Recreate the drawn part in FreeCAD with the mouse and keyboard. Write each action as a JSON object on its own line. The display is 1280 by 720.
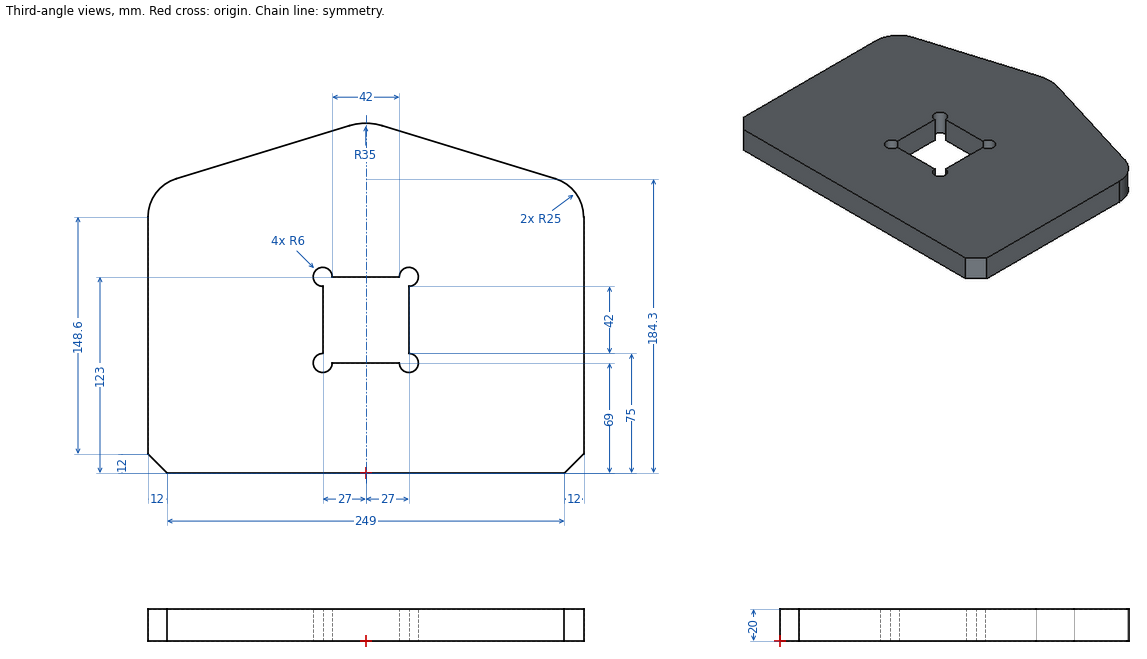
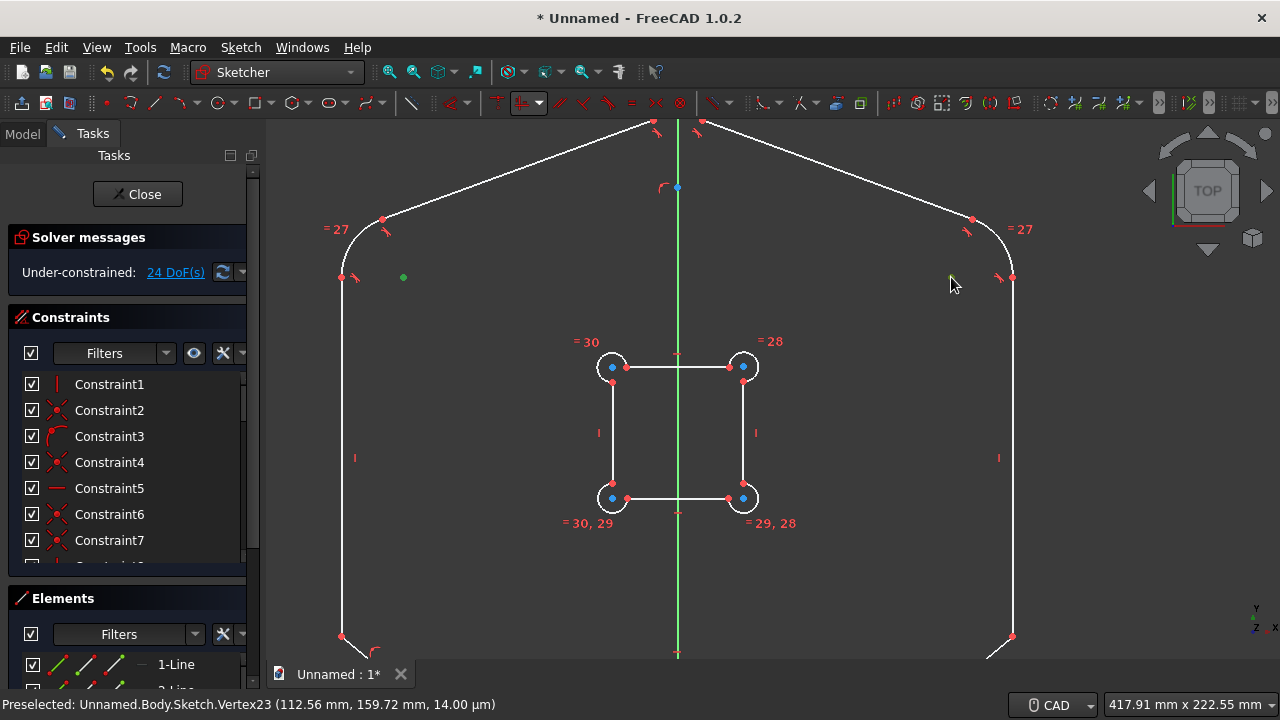
{"action": "left_click", "coordinate": [678, 596]}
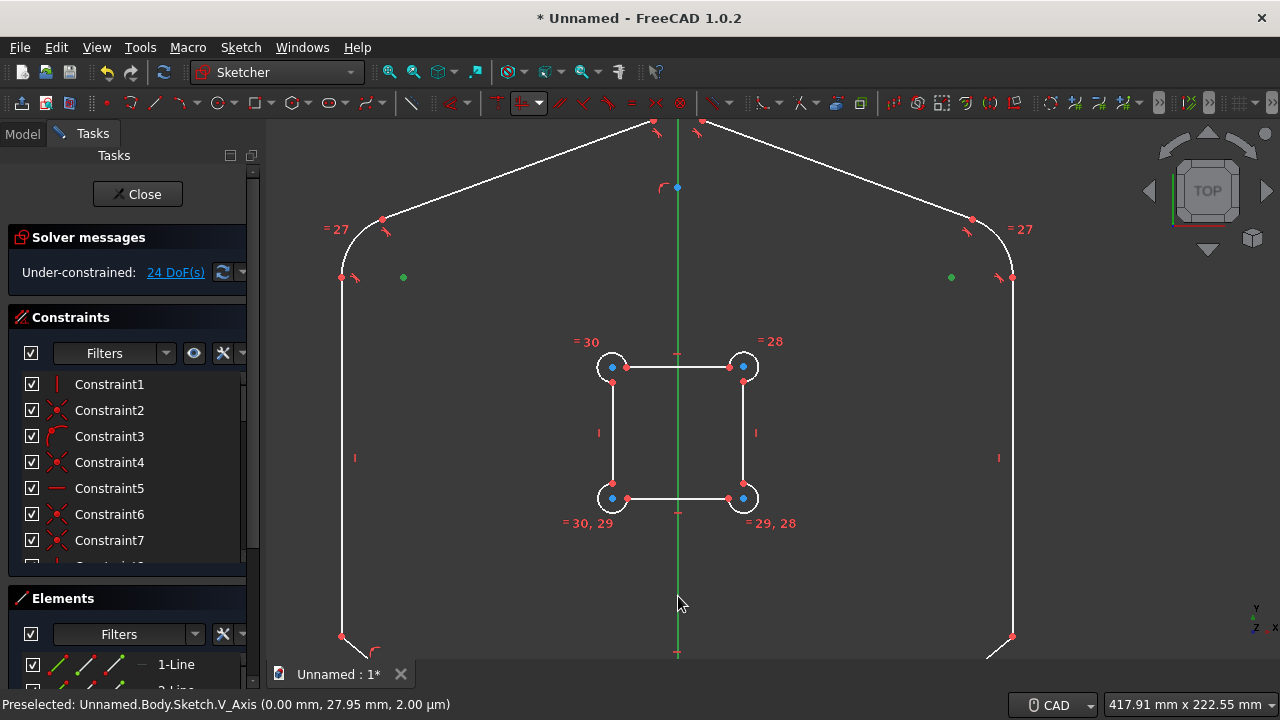
{"action": "left_click", "coordinate": [656, 104]}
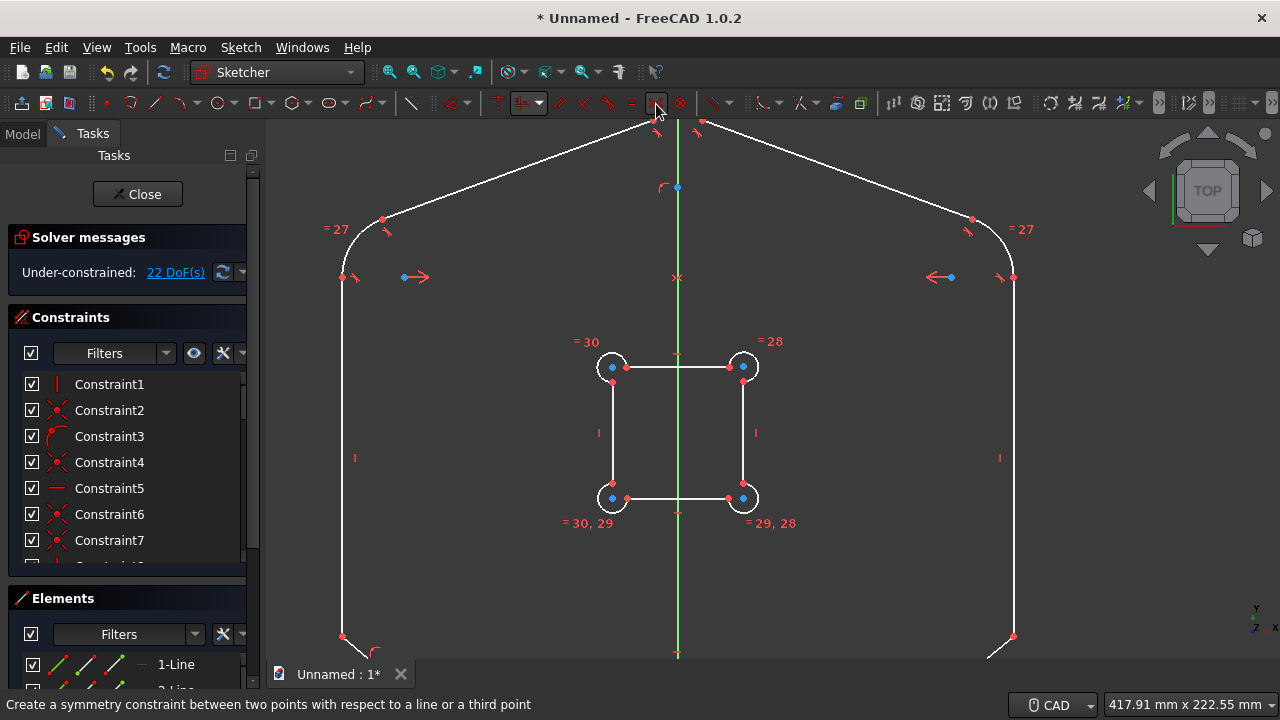
{"action": "left_click", "coordinate": [744, 498]}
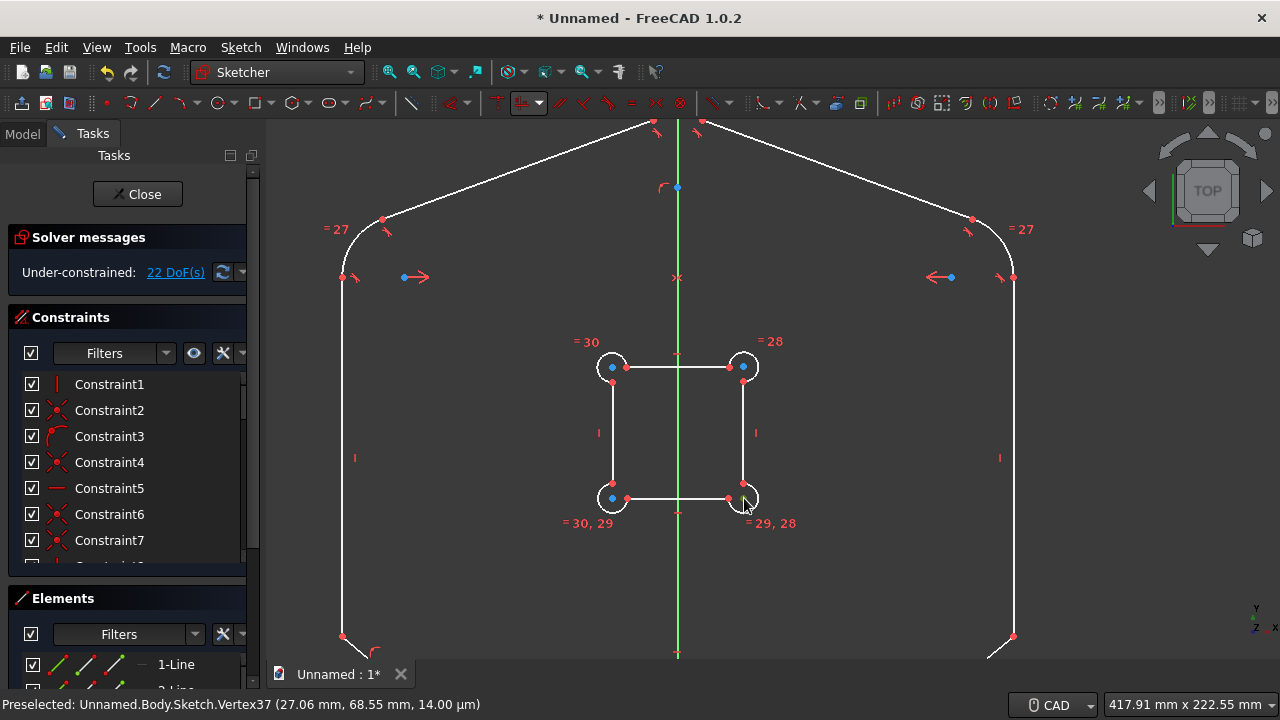
{"action": "left_click", "coordinate": [613, 498]}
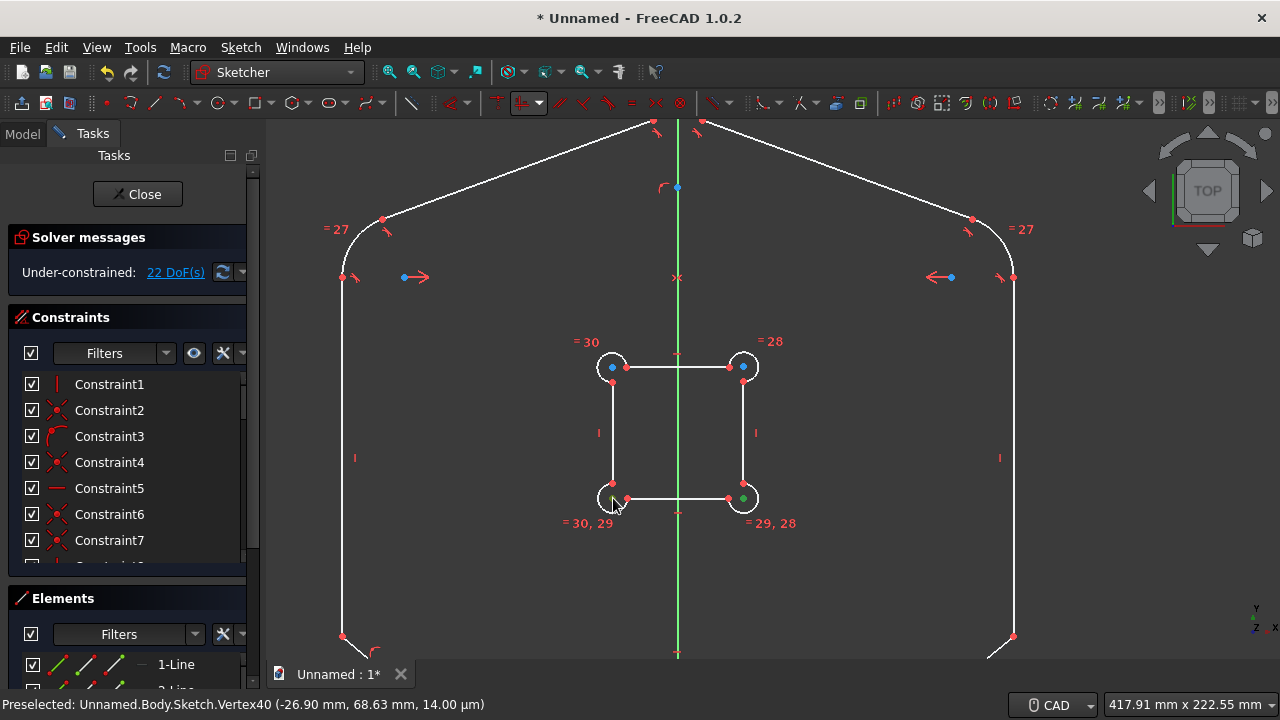
{"action": "left_click", "coordinate": [678, 596]}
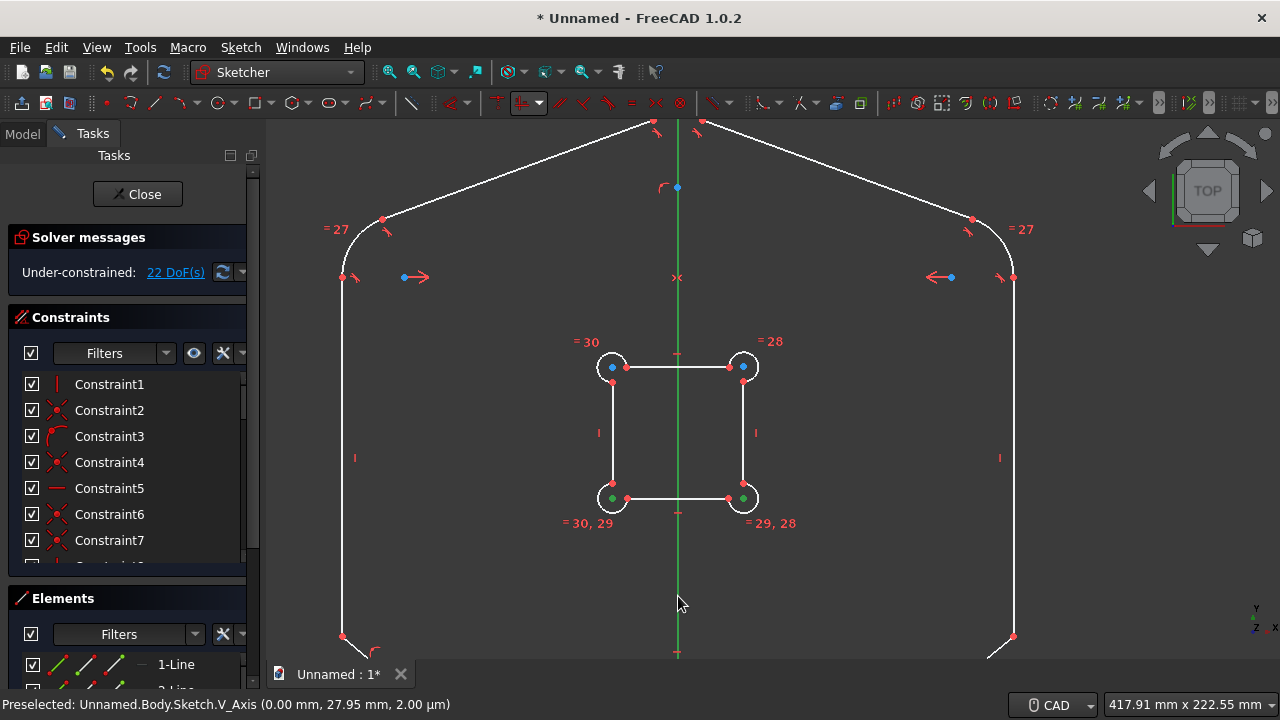
{"action": "left_click", "coordinate": [656, 104]}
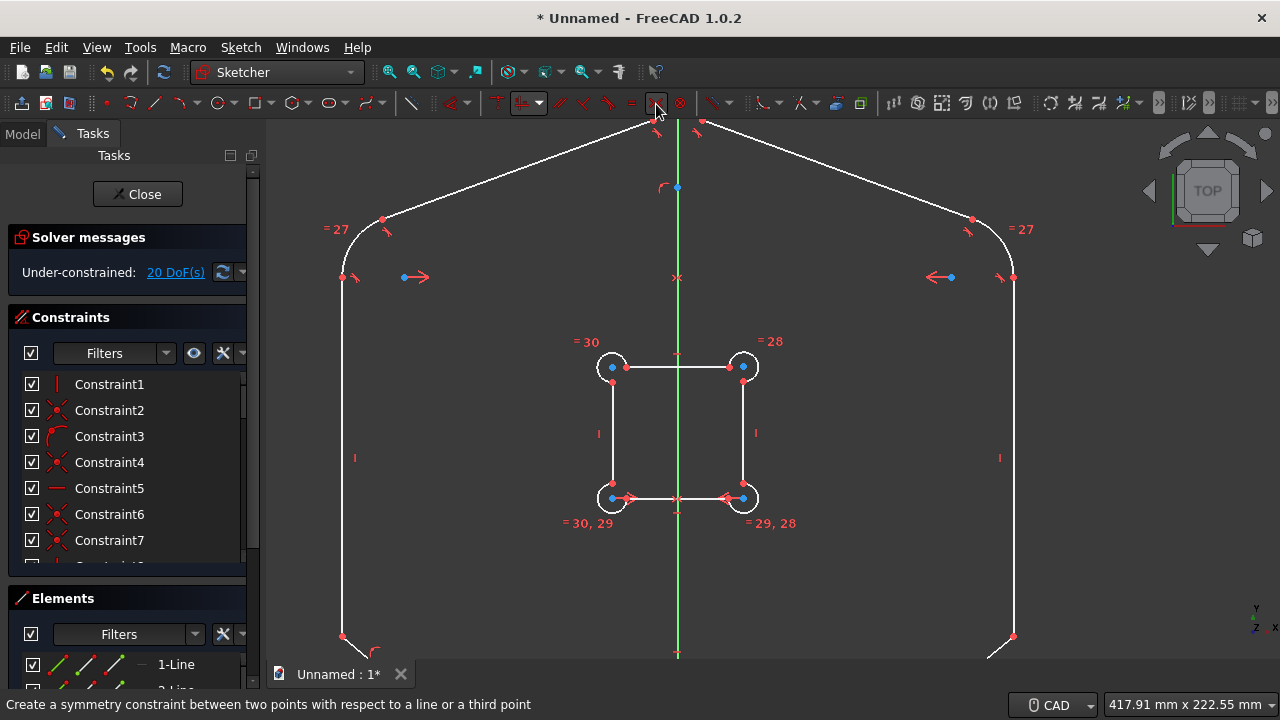
{"action": "left_click", "coordinate": [744, 367]}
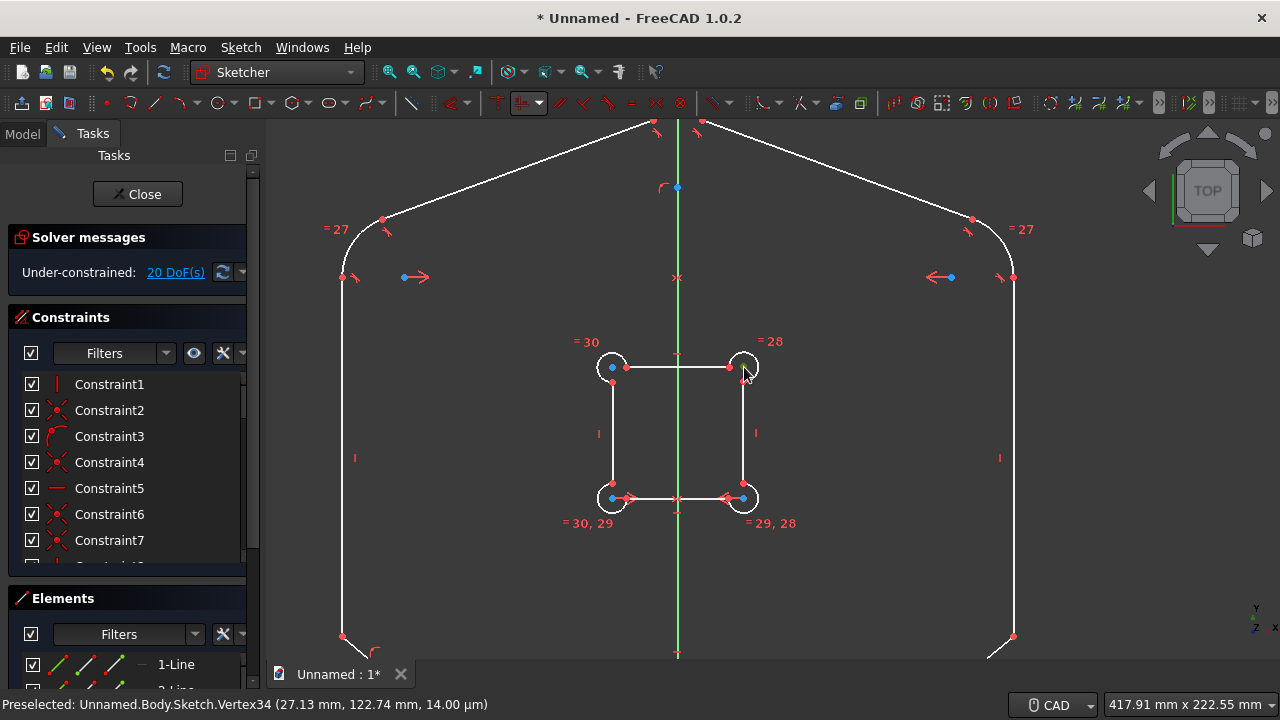
{"action": "left_click", "coordinate": [612, 368]}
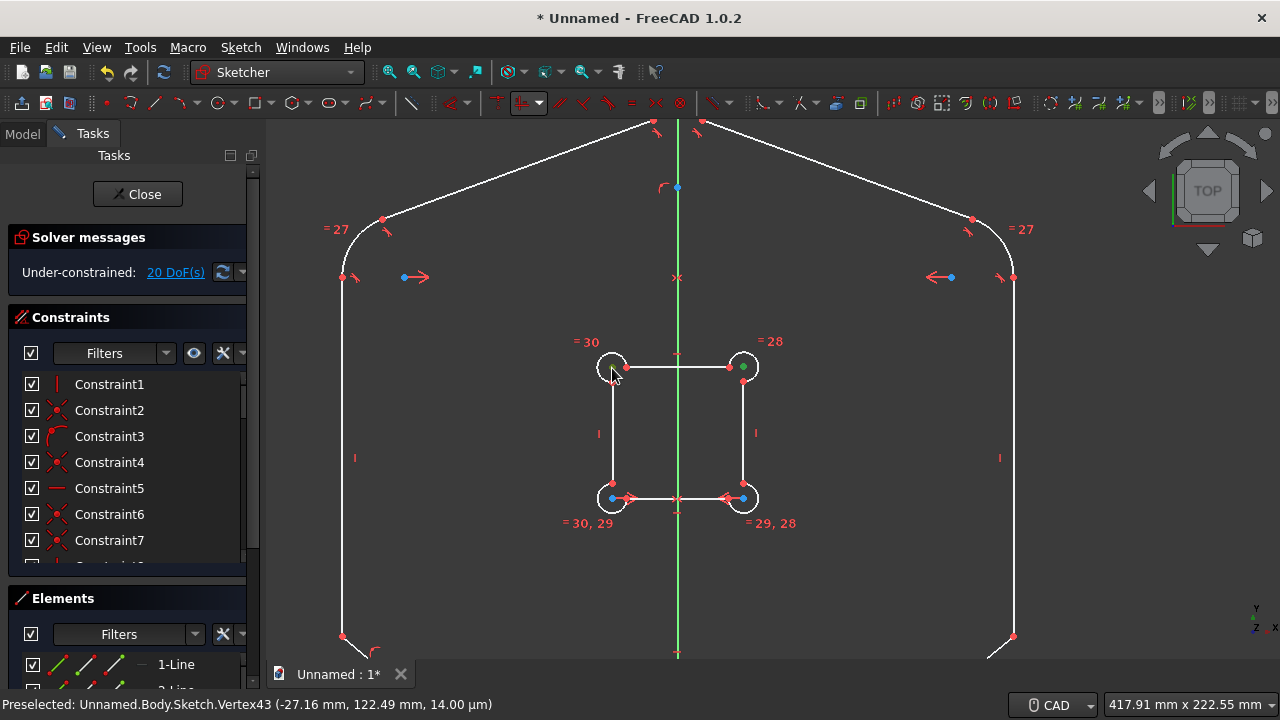
{"action": "left_click", "coordinate": [678, 596]}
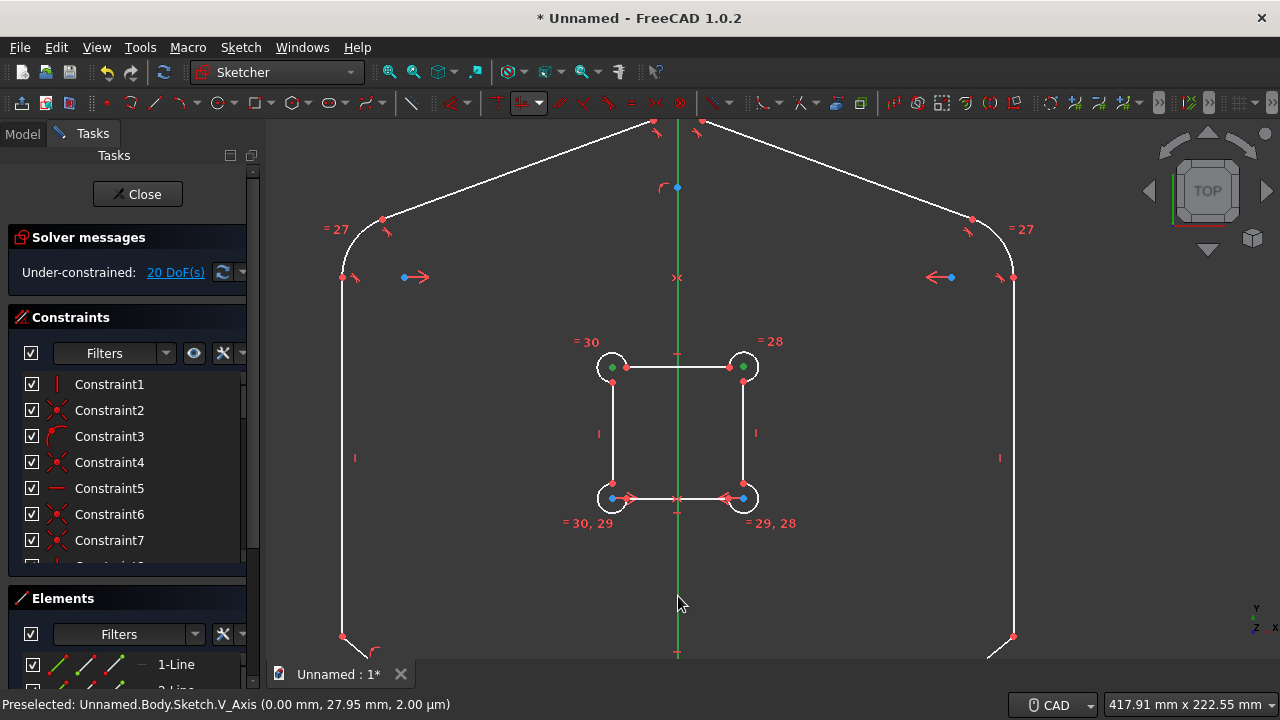
{"action": "left_click", "coordinate": [656, 104]}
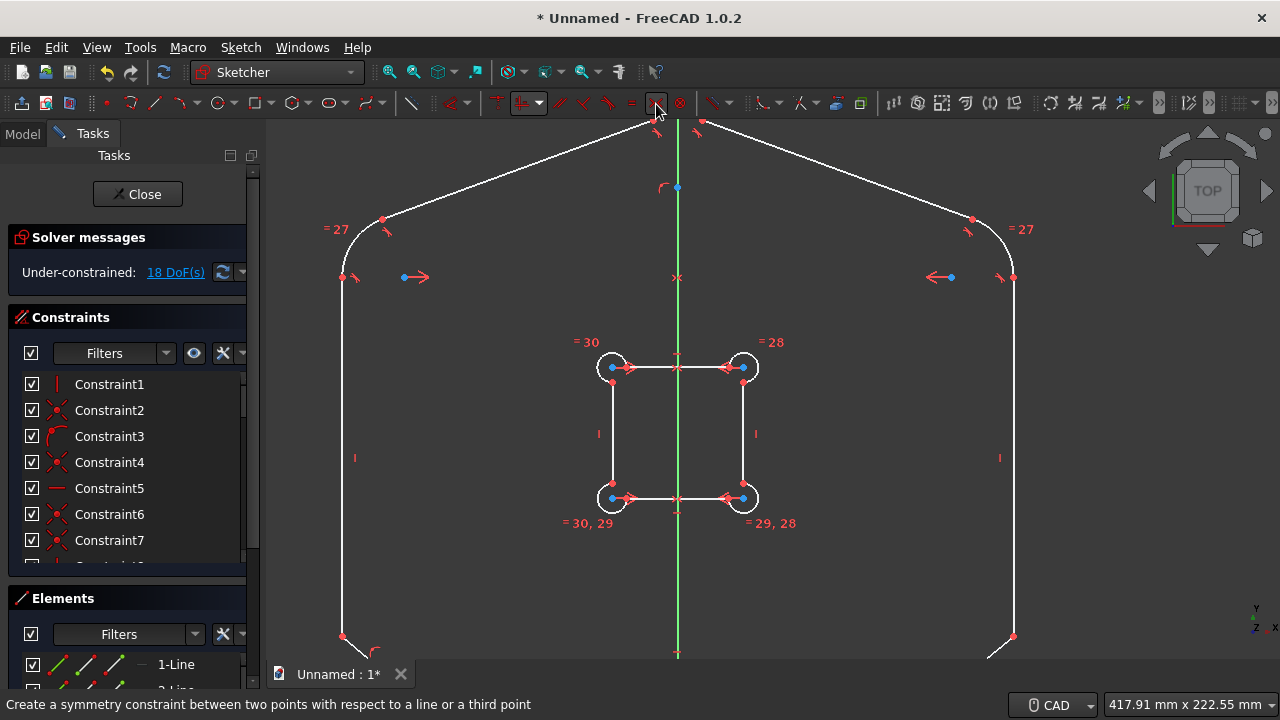
{"action": "left_click", "coordinate": [450, 104]}